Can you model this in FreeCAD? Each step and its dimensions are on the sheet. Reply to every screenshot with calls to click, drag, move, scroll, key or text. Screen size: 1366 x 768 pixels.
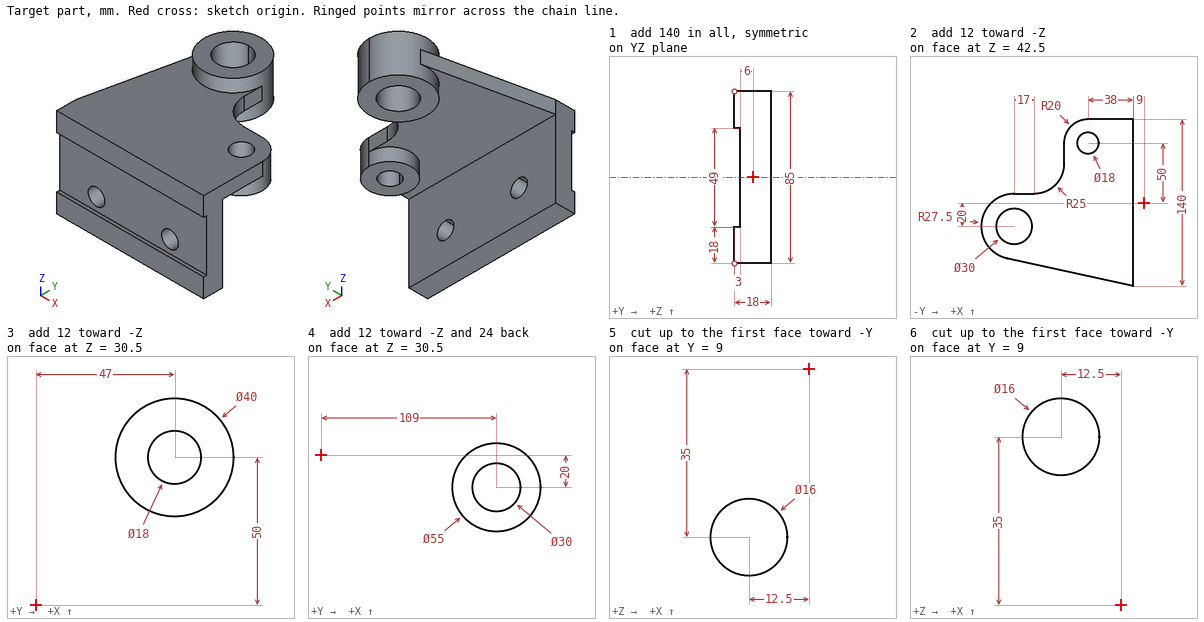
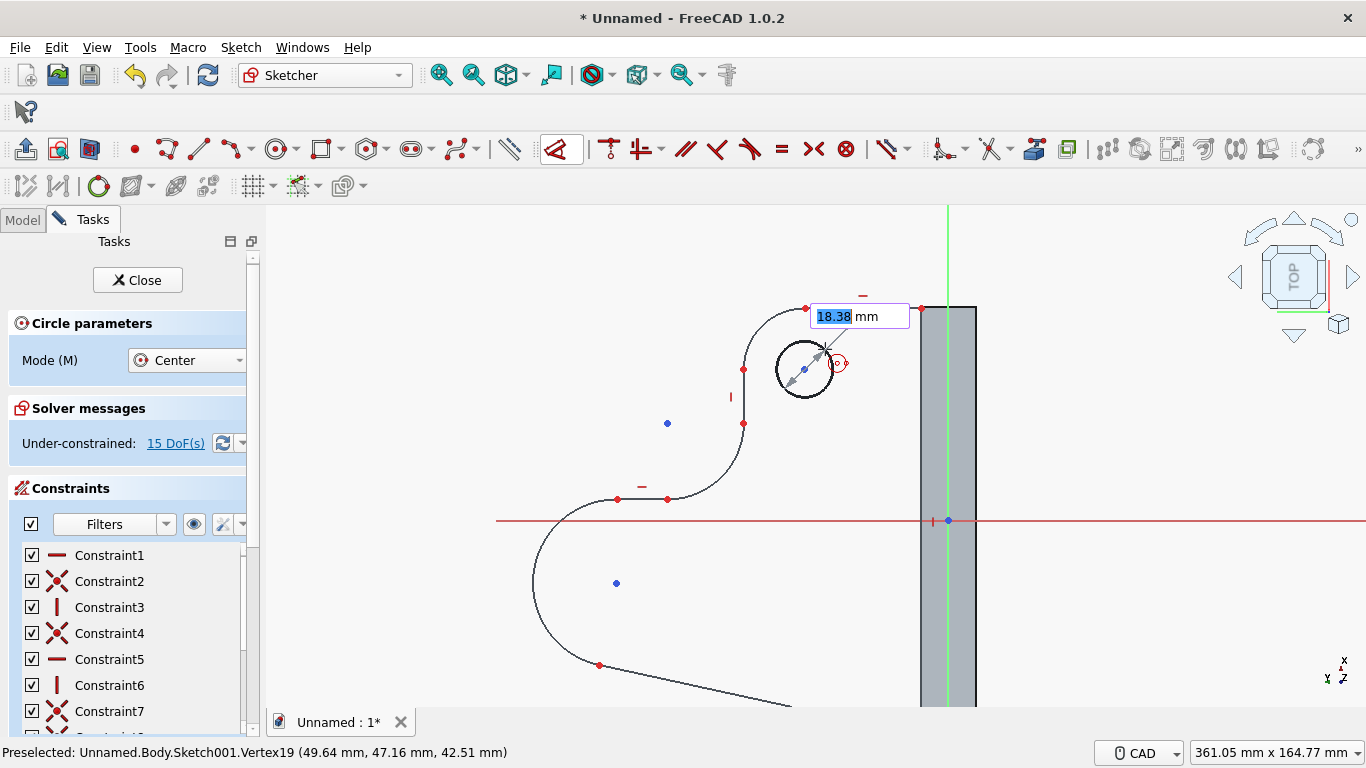
text(18)
key(Return)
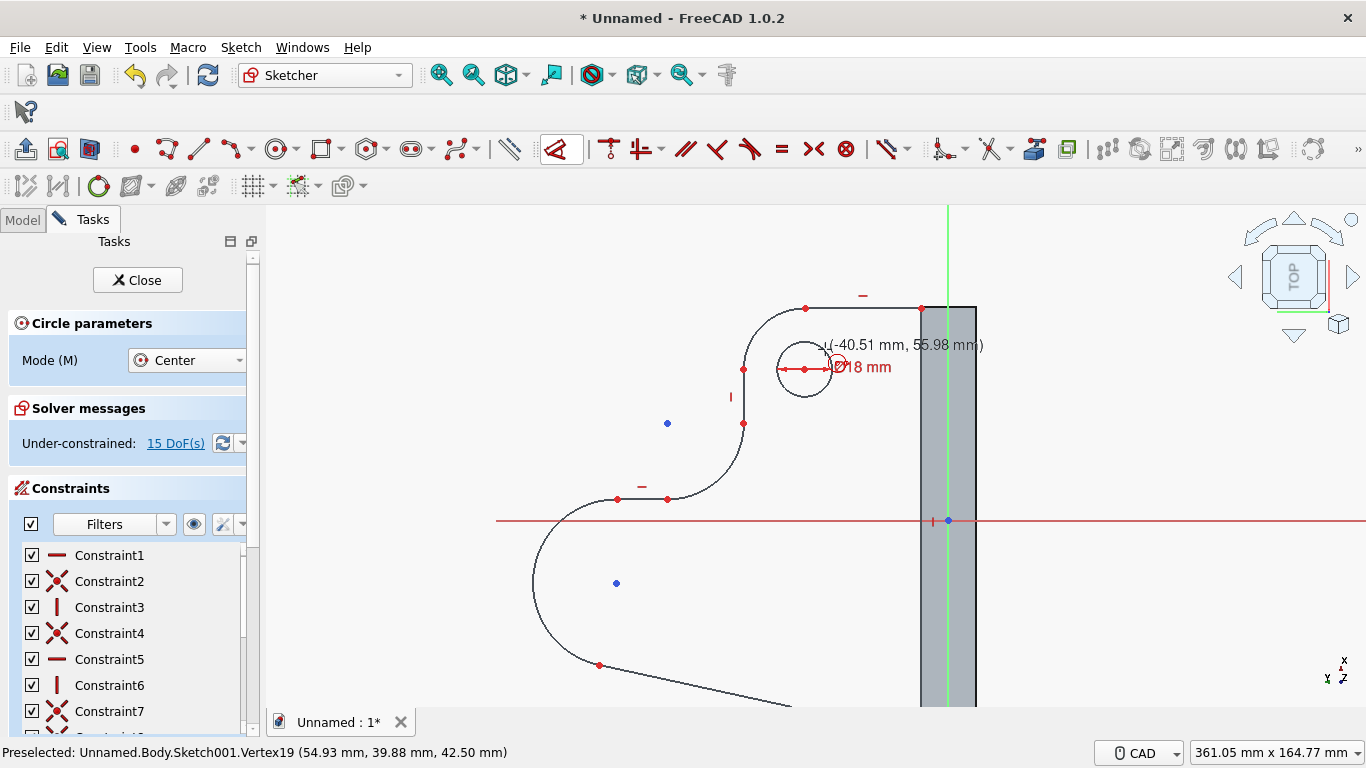
click(616, 581)
move(649, 549)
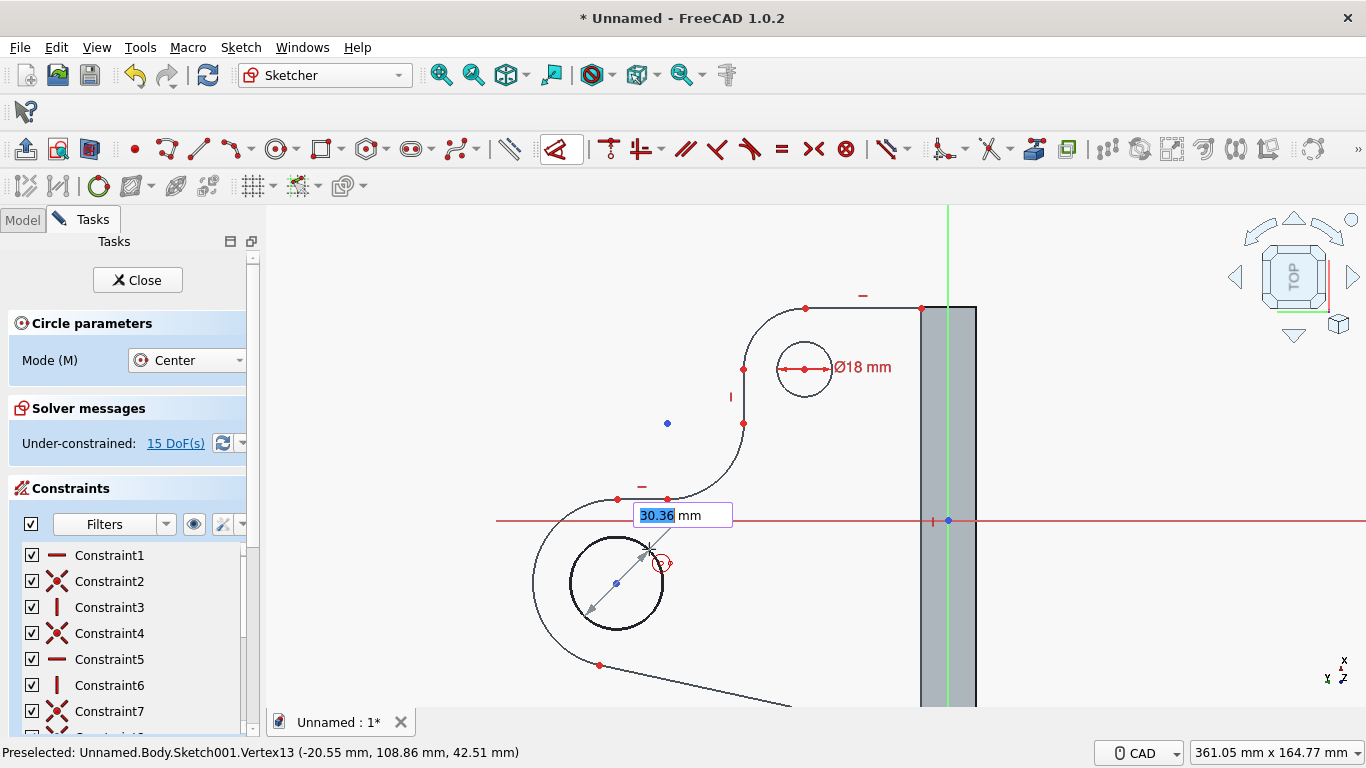
text(30)
key(Return)
key(Escape)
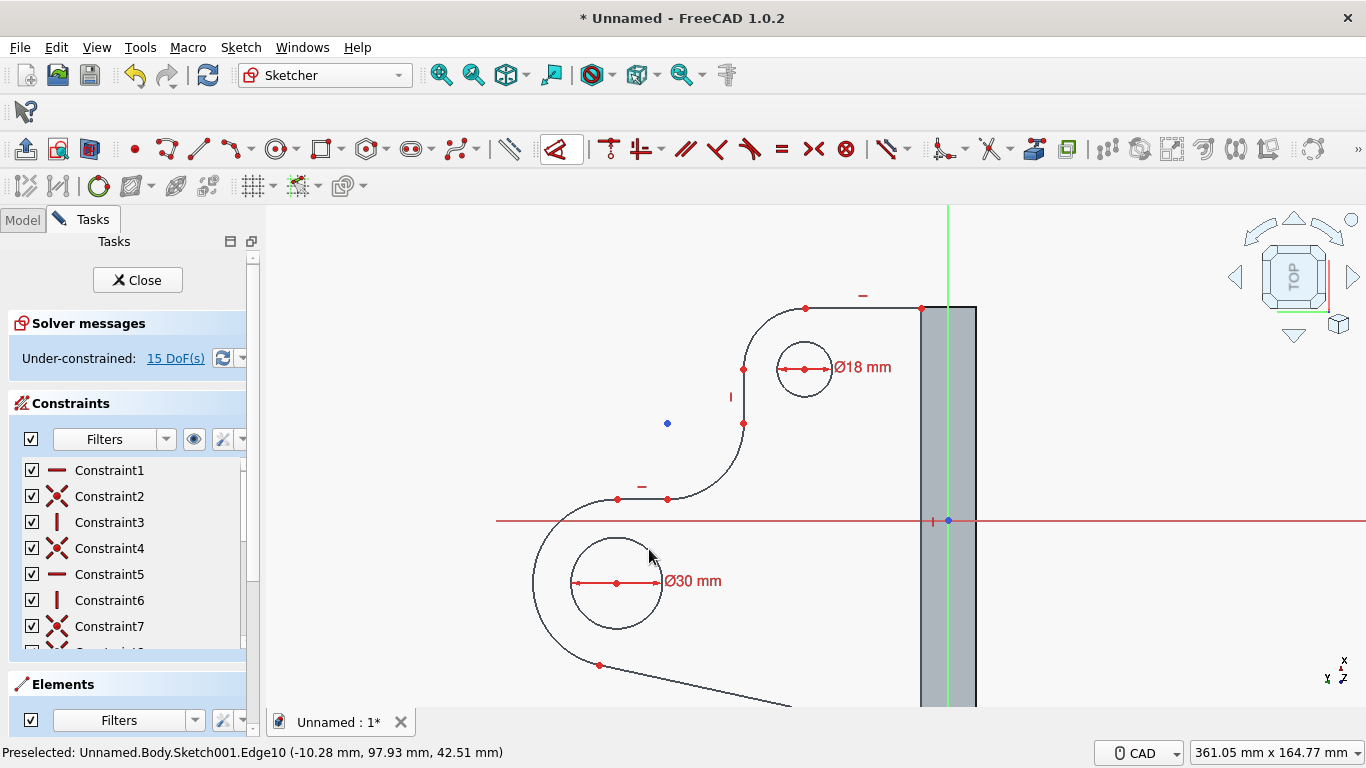
click(840, 308)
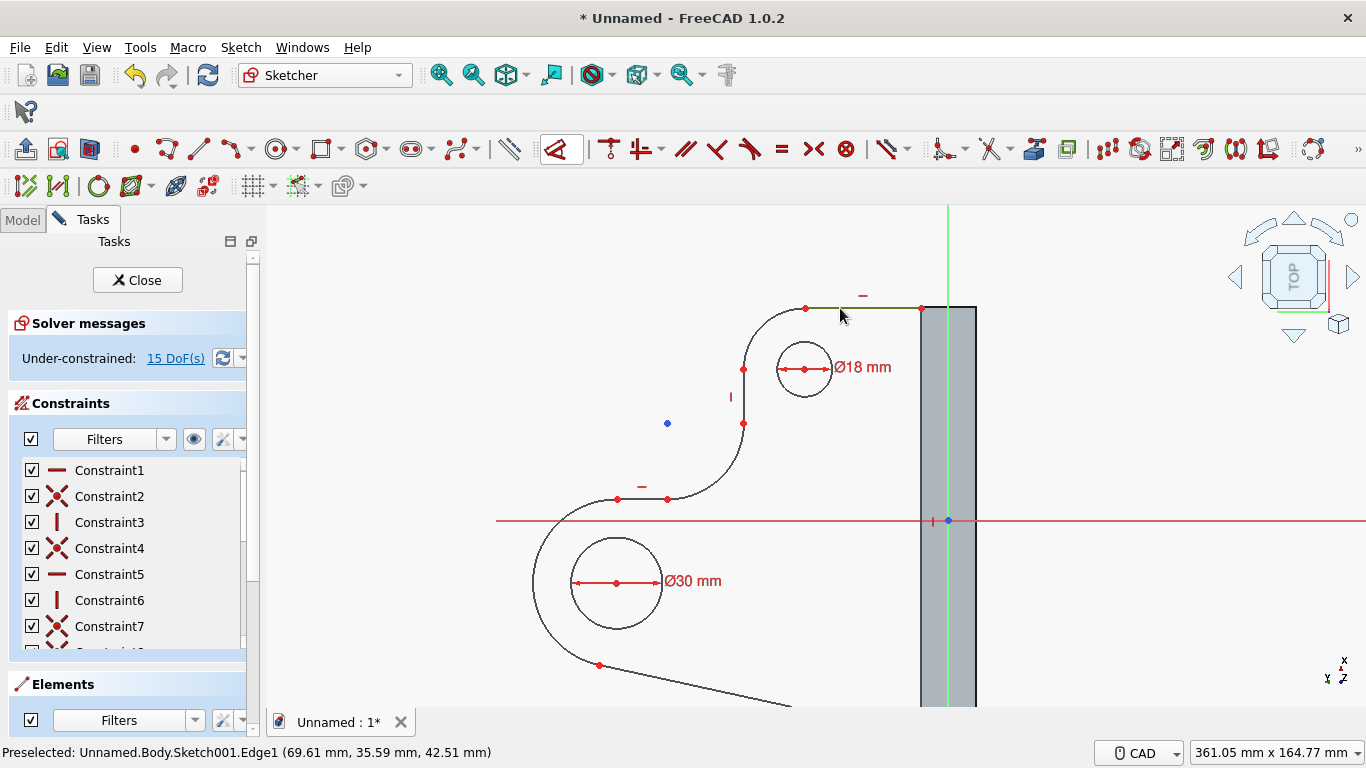
click(777, 315)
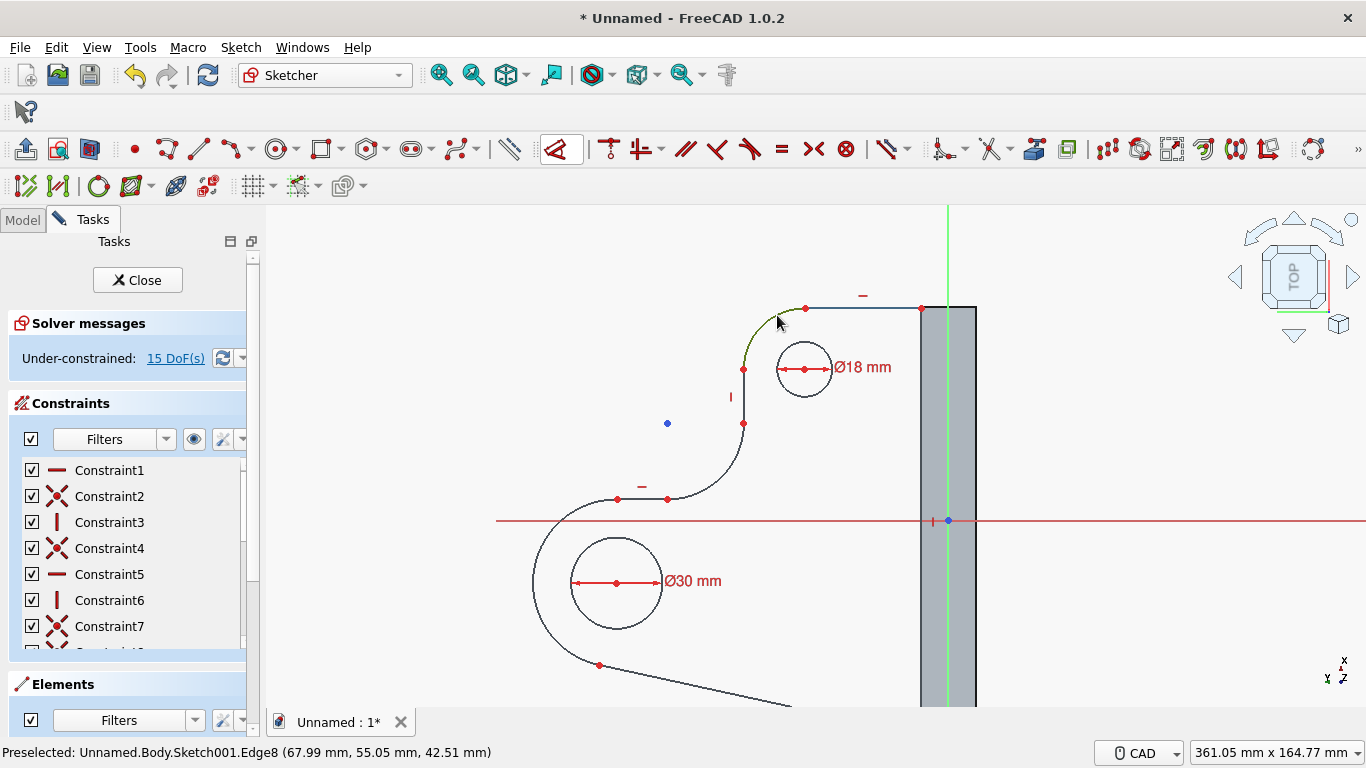
key(t)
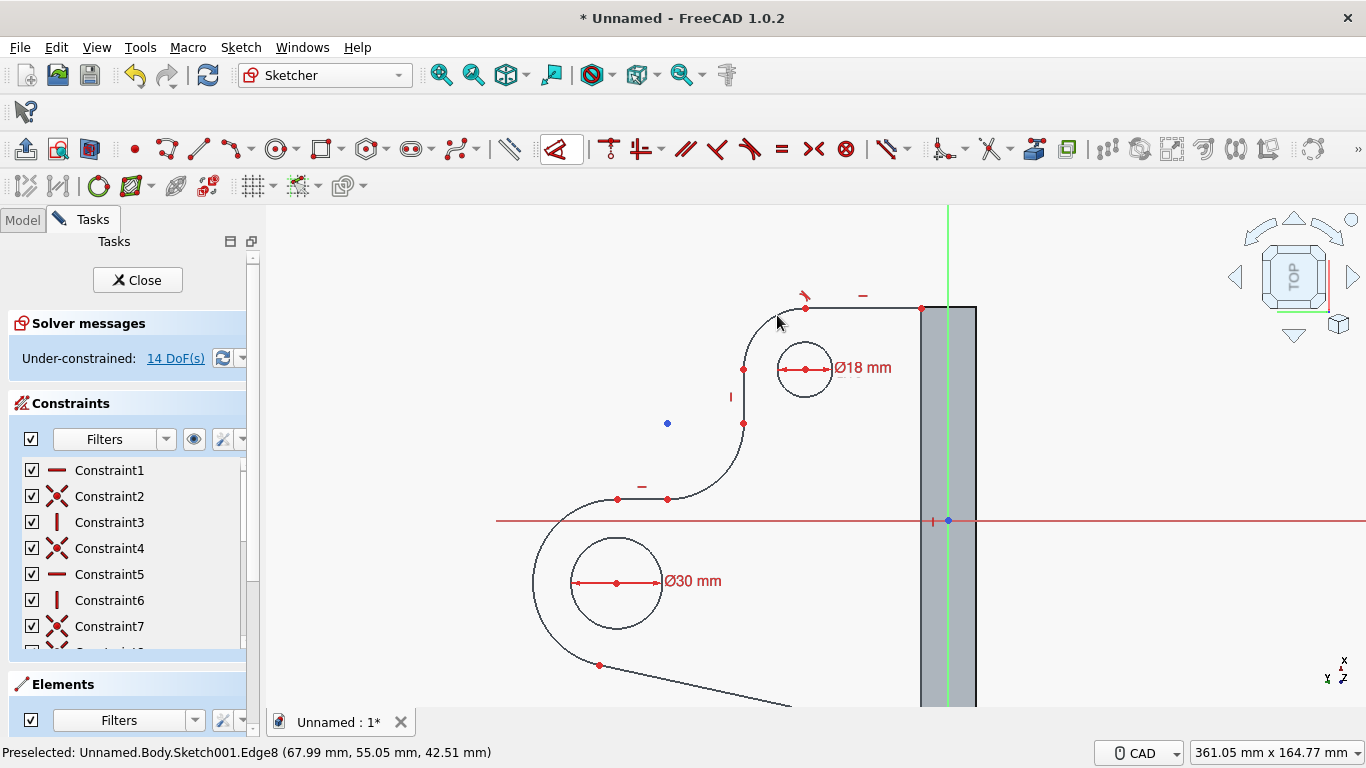
scroll(761, 325, down, 2)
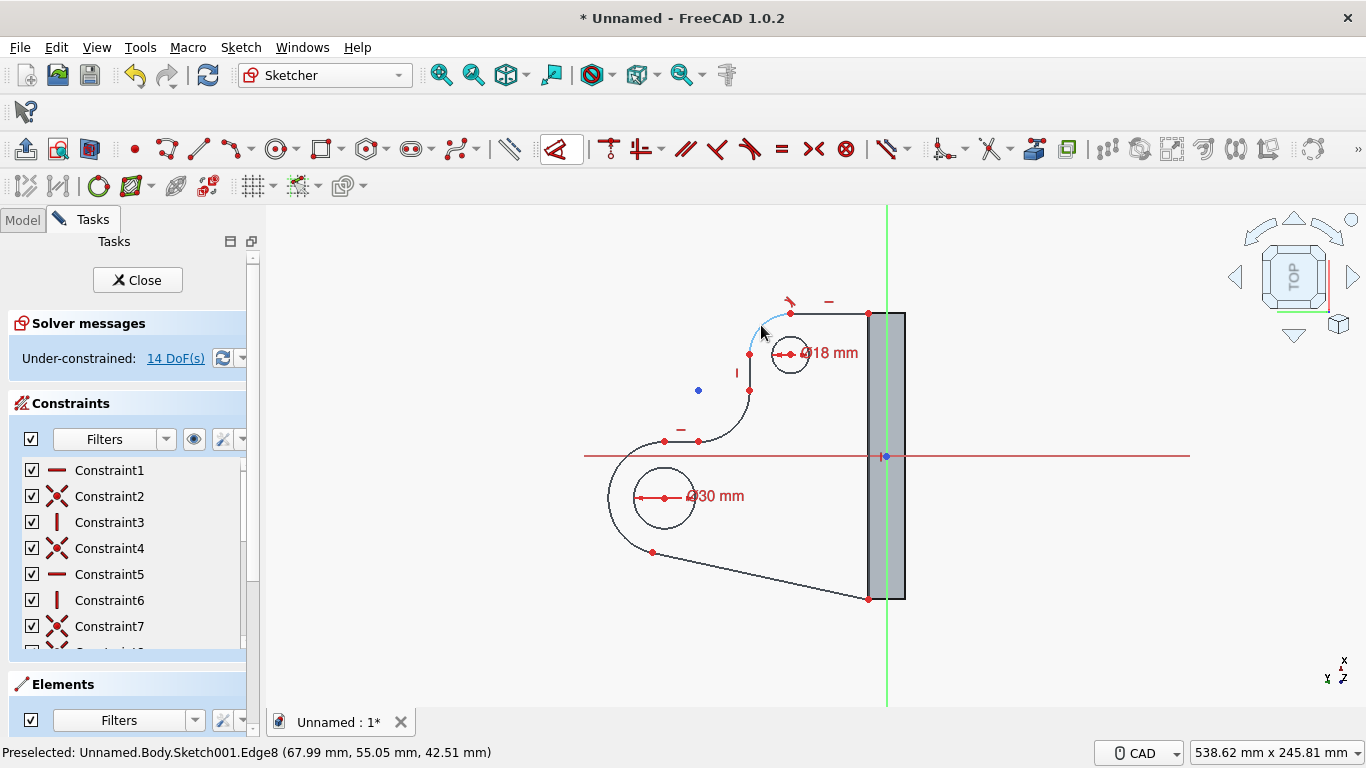
click(804, 586)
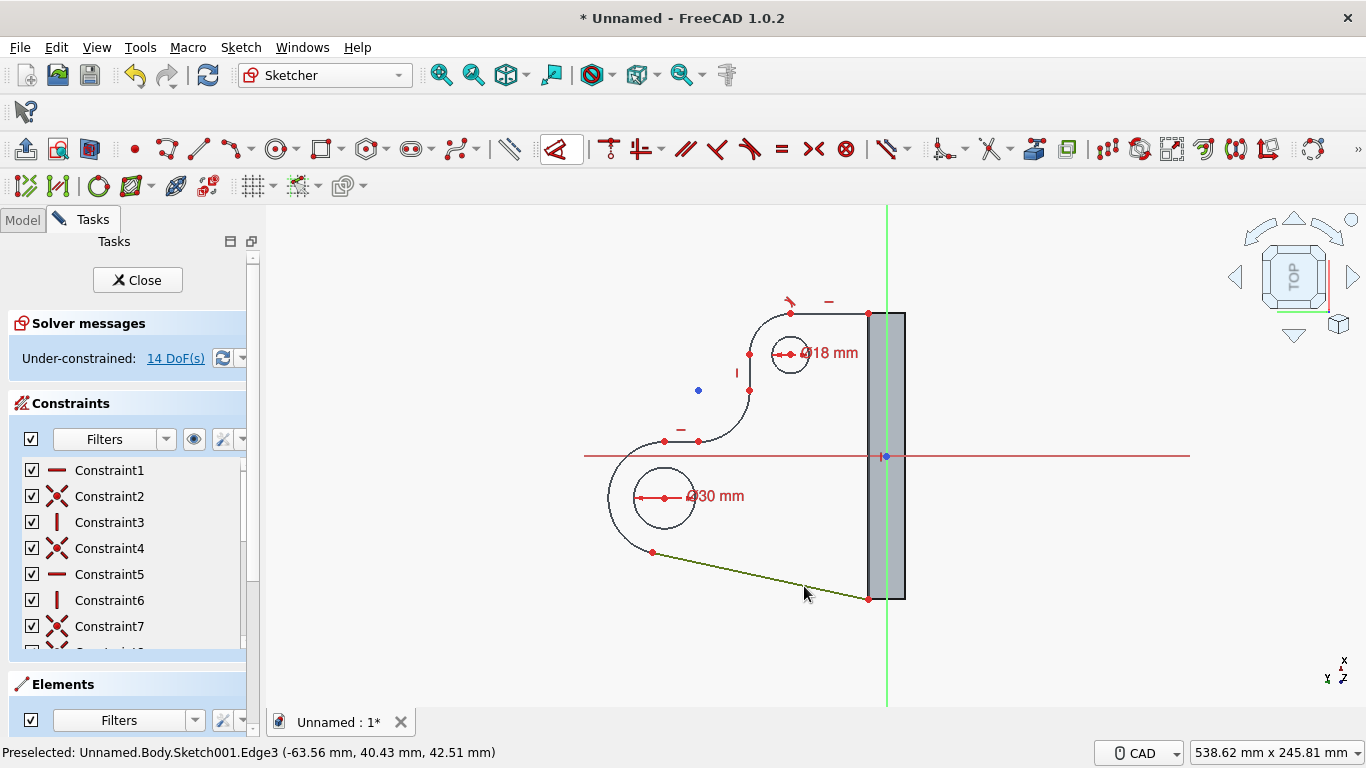
click(615, 524)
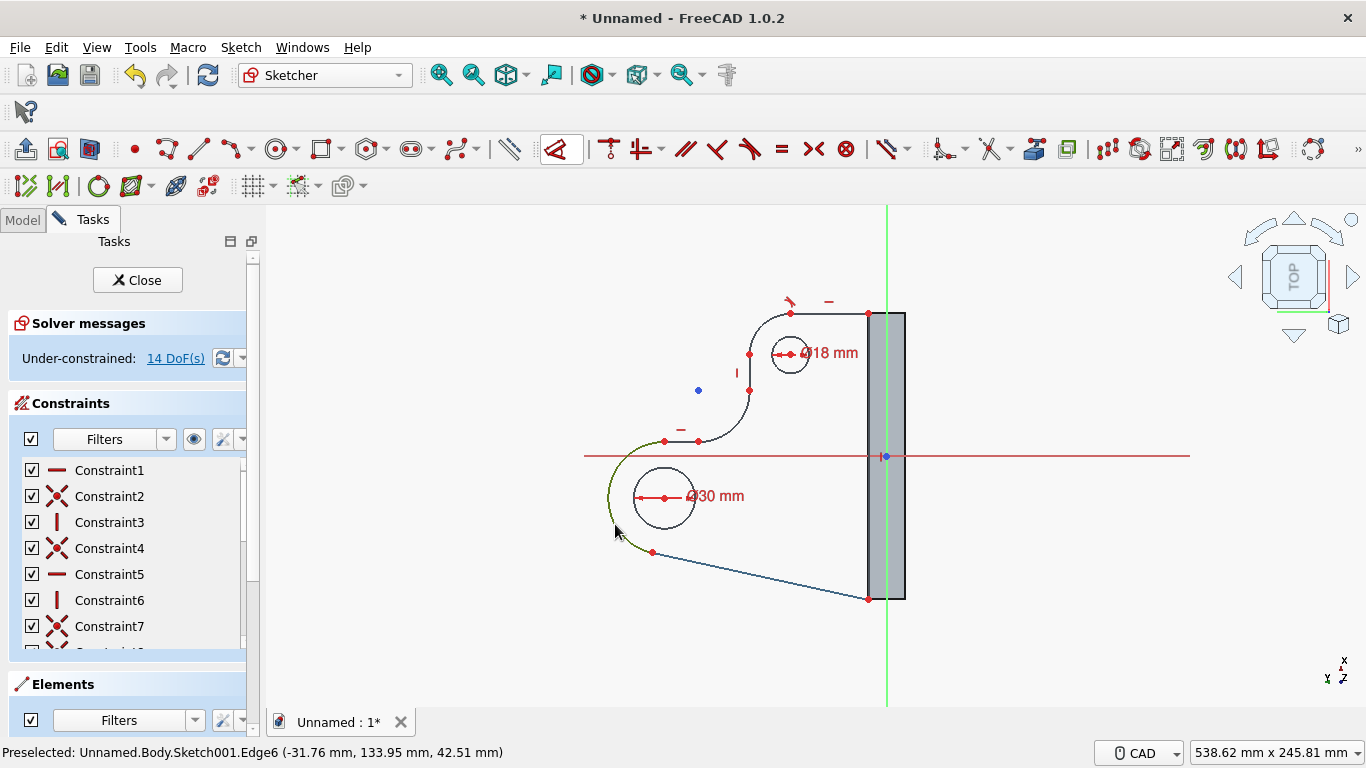
click(750, 150)